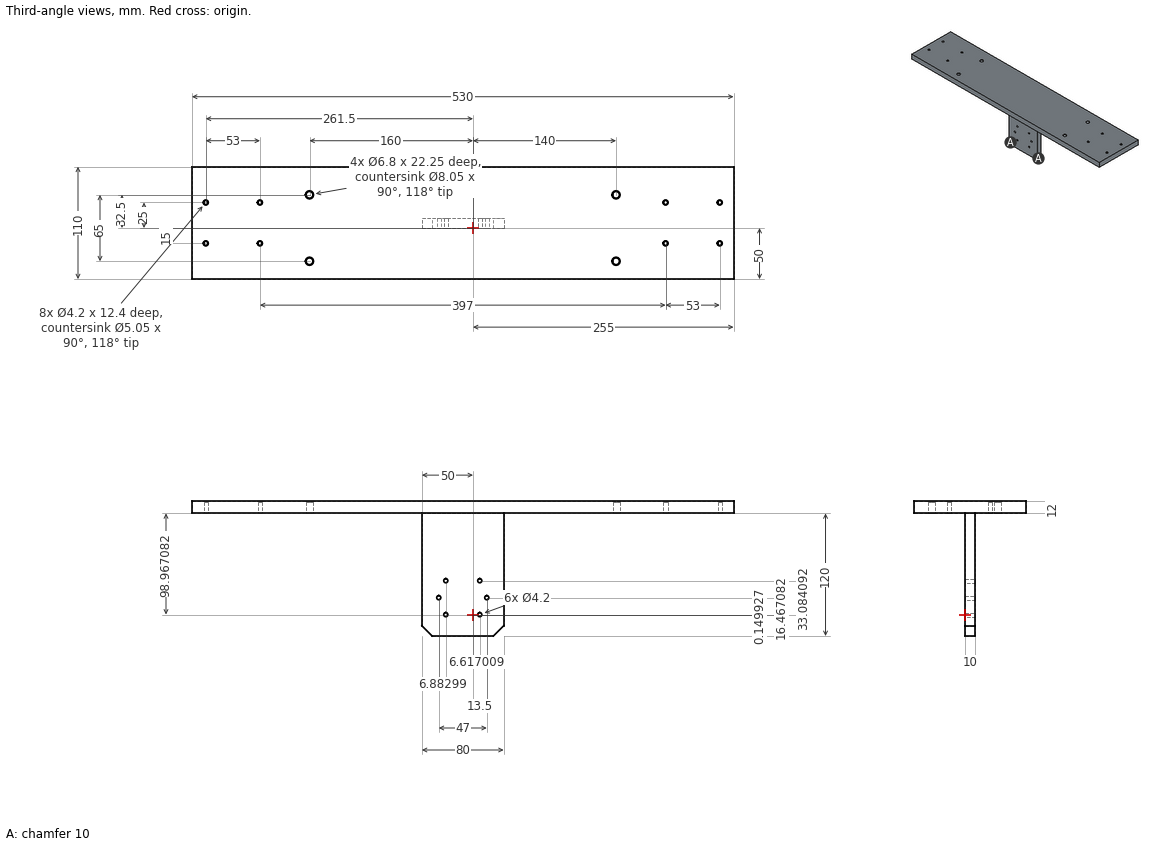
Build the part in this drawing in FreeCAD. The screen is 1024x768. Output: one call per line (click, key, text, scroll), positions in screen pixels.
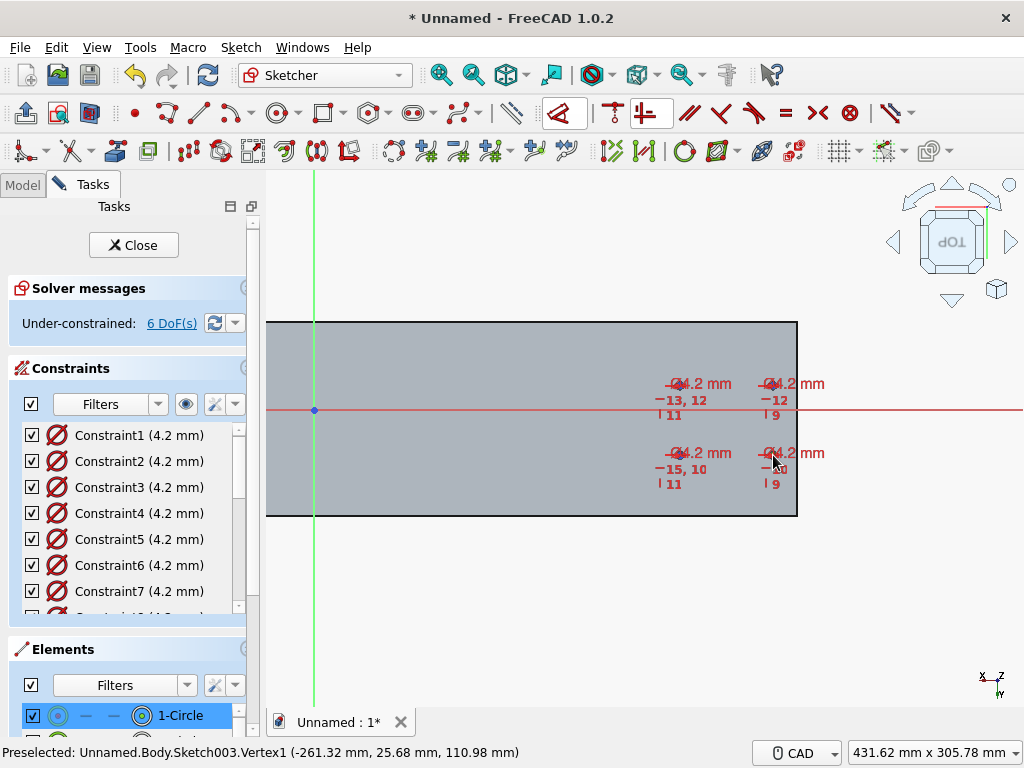
key(i)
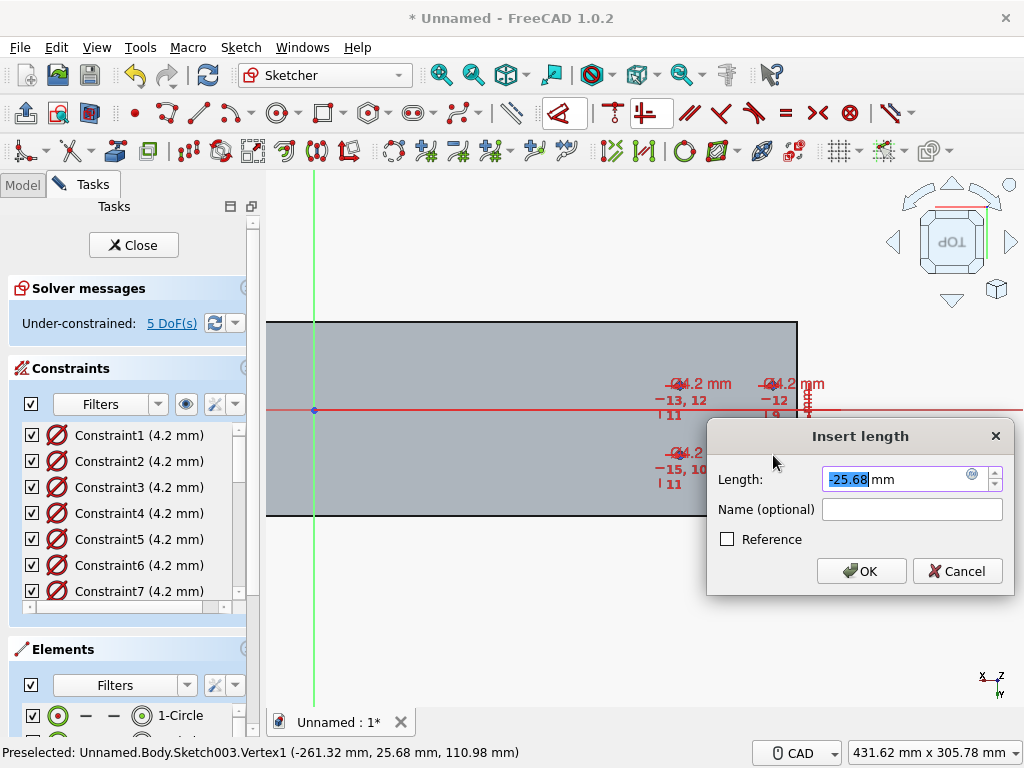
text(-25)
key(Return)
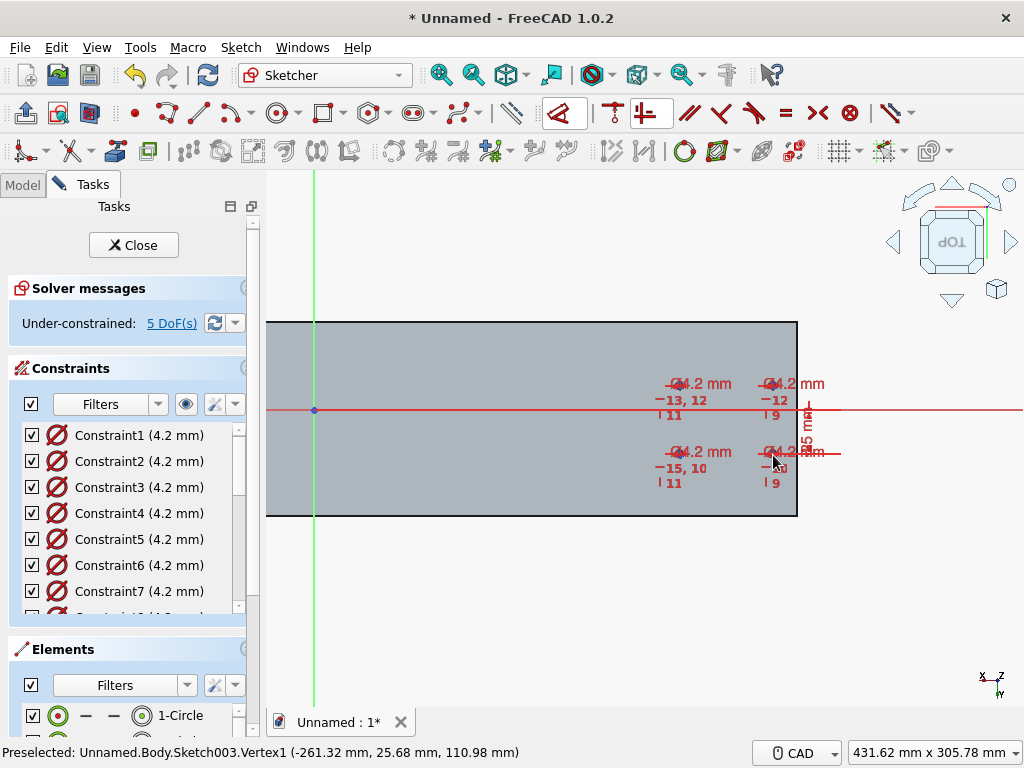
scroll(773, 386, up, 3)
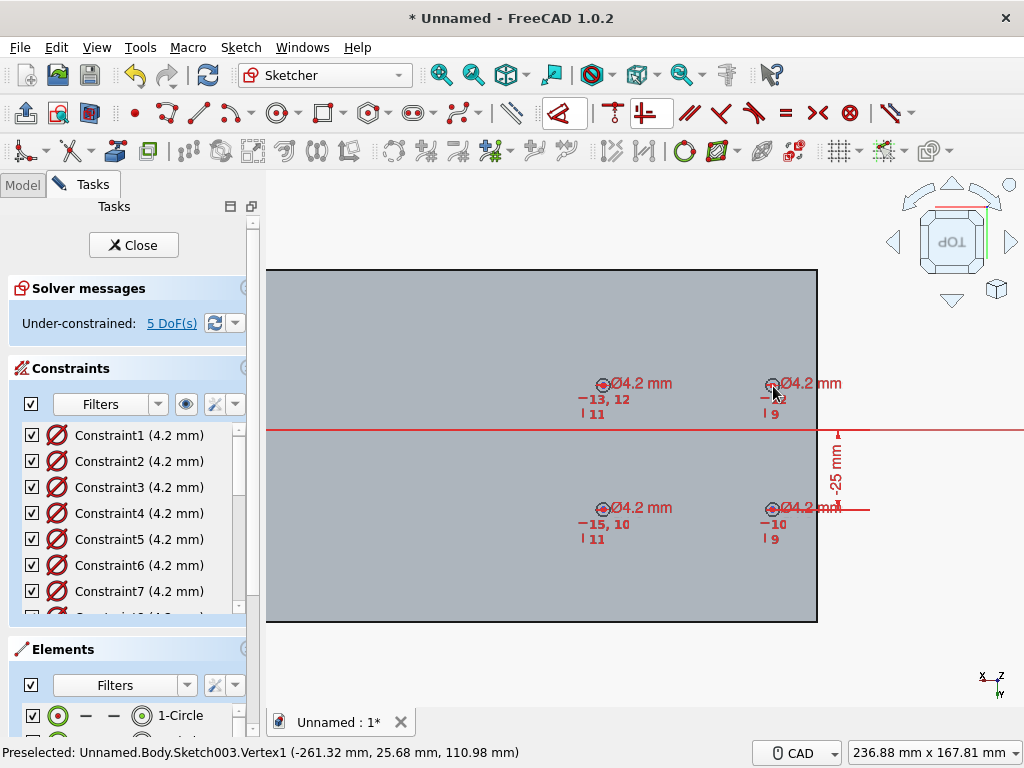
click(773, 385)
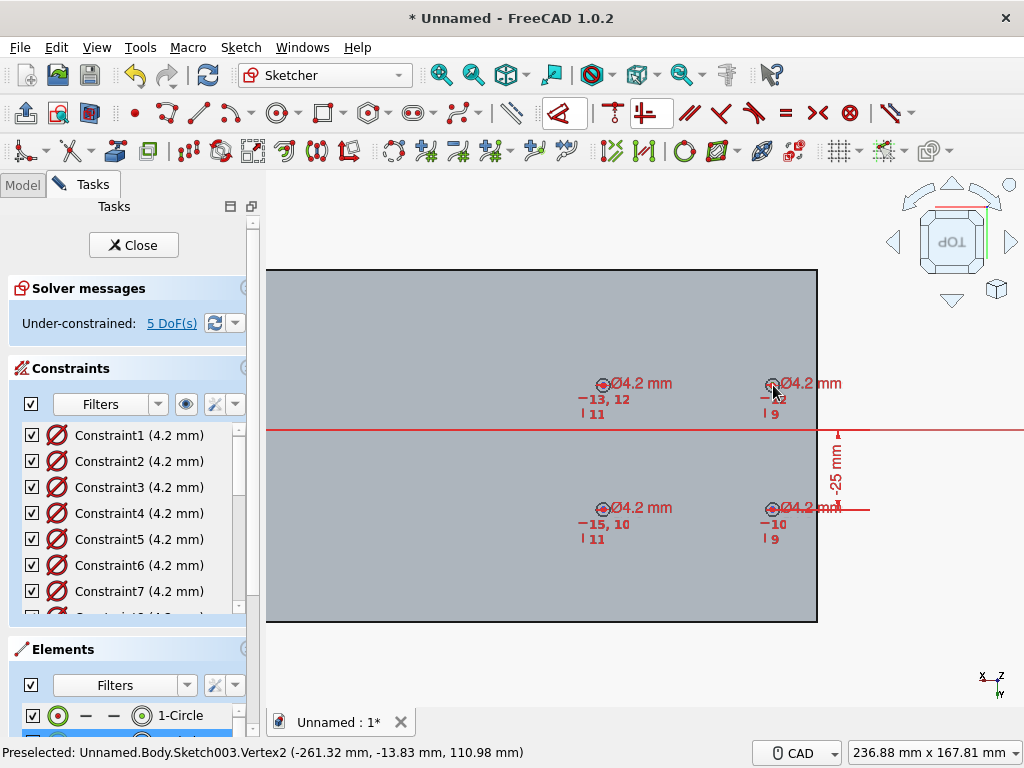
key(i)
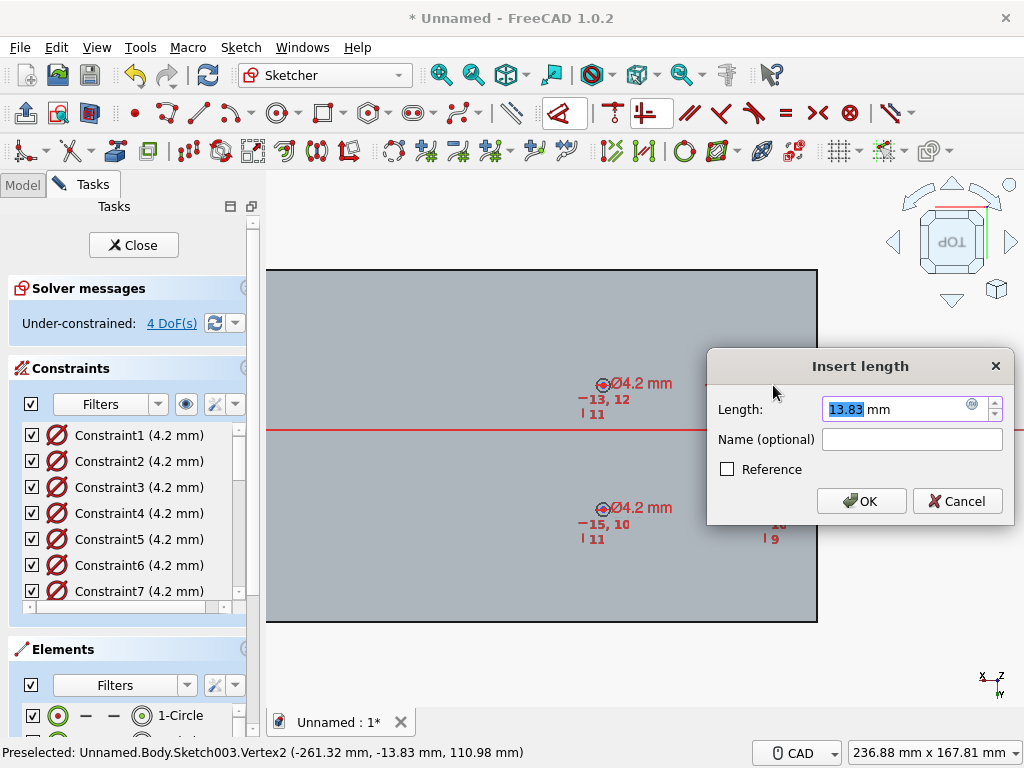
text(15)
key(Return)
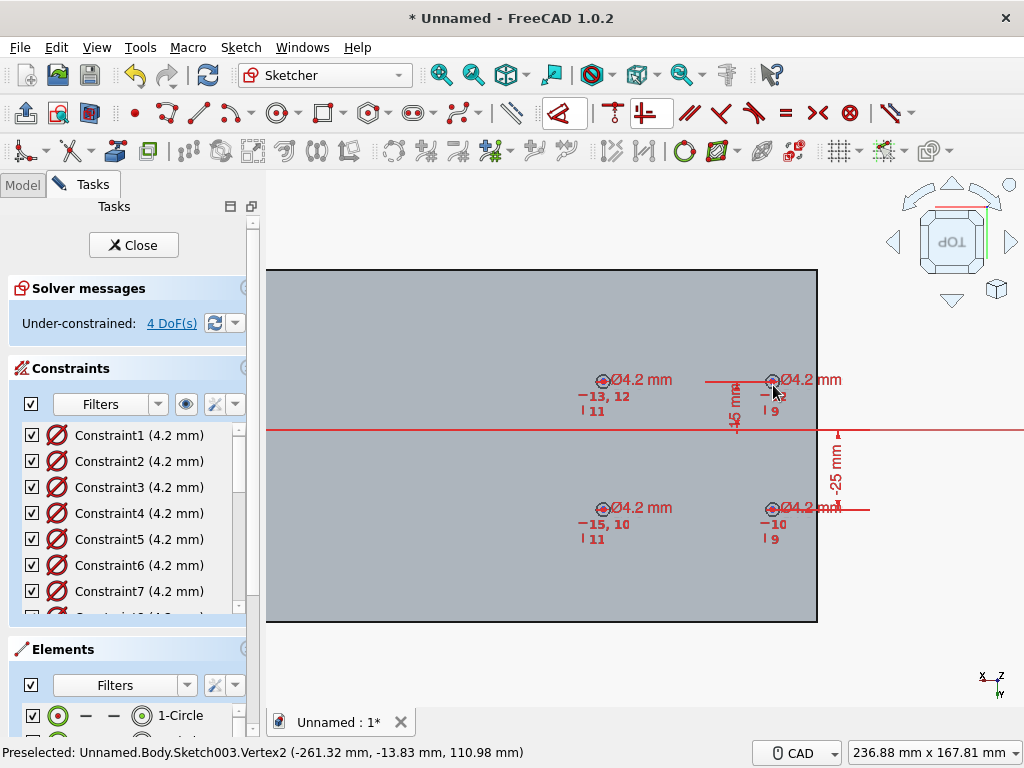
scroll(775, 436, down, 7)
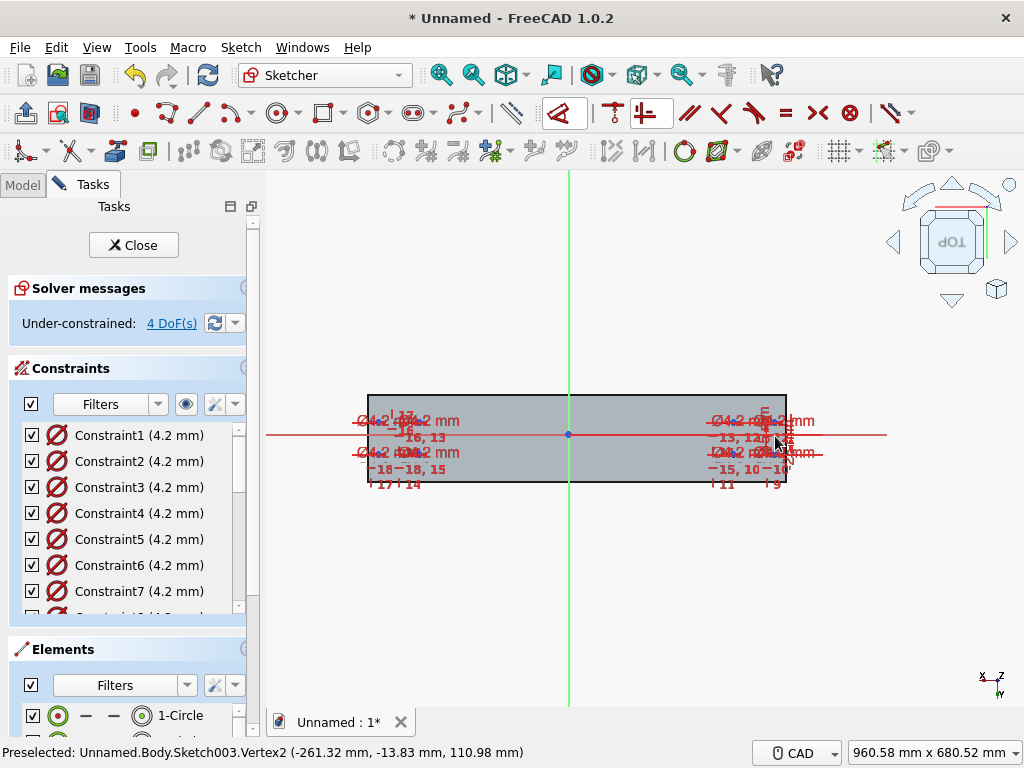
click(775, 455)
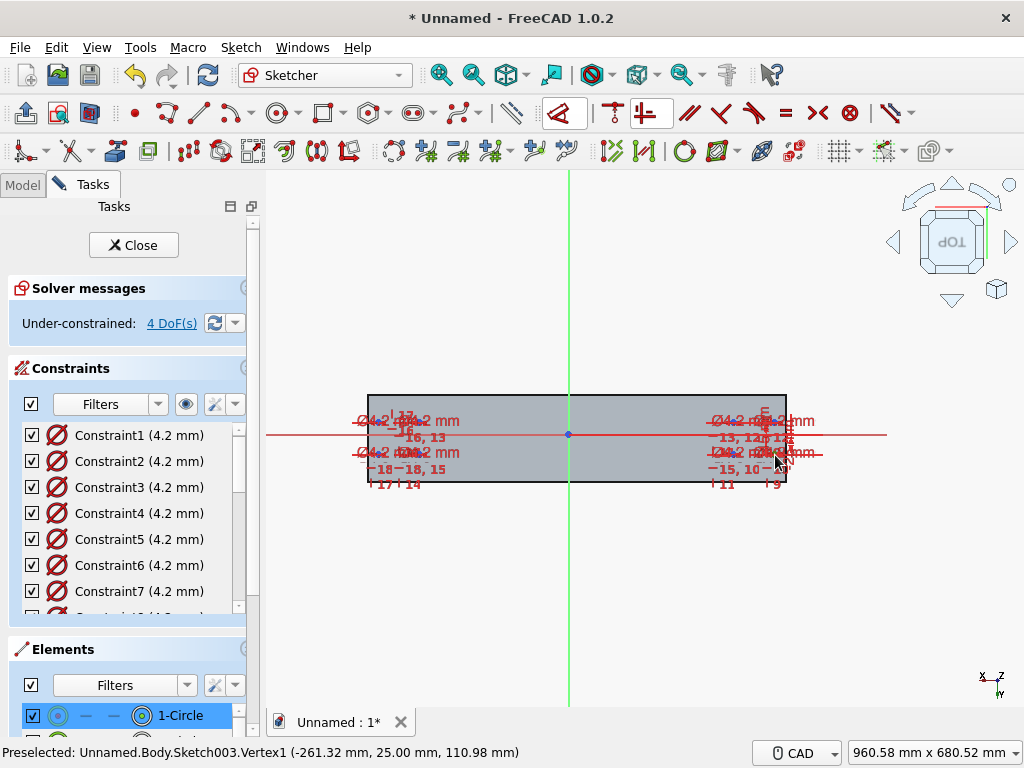
click(733, 455)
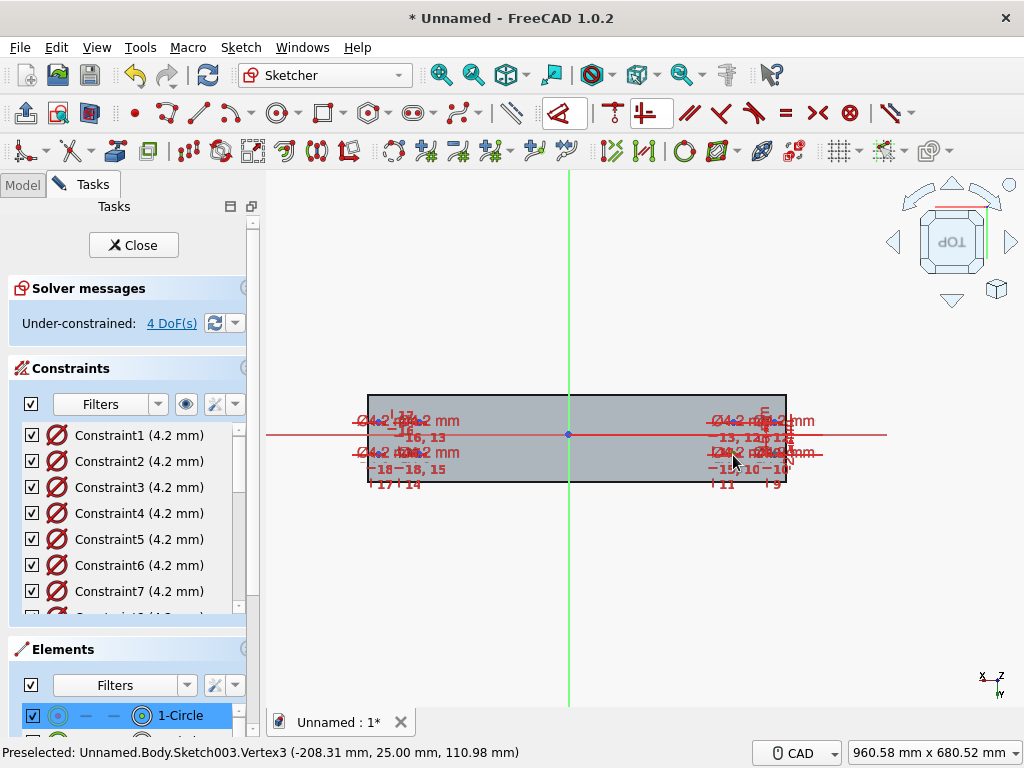
key(l)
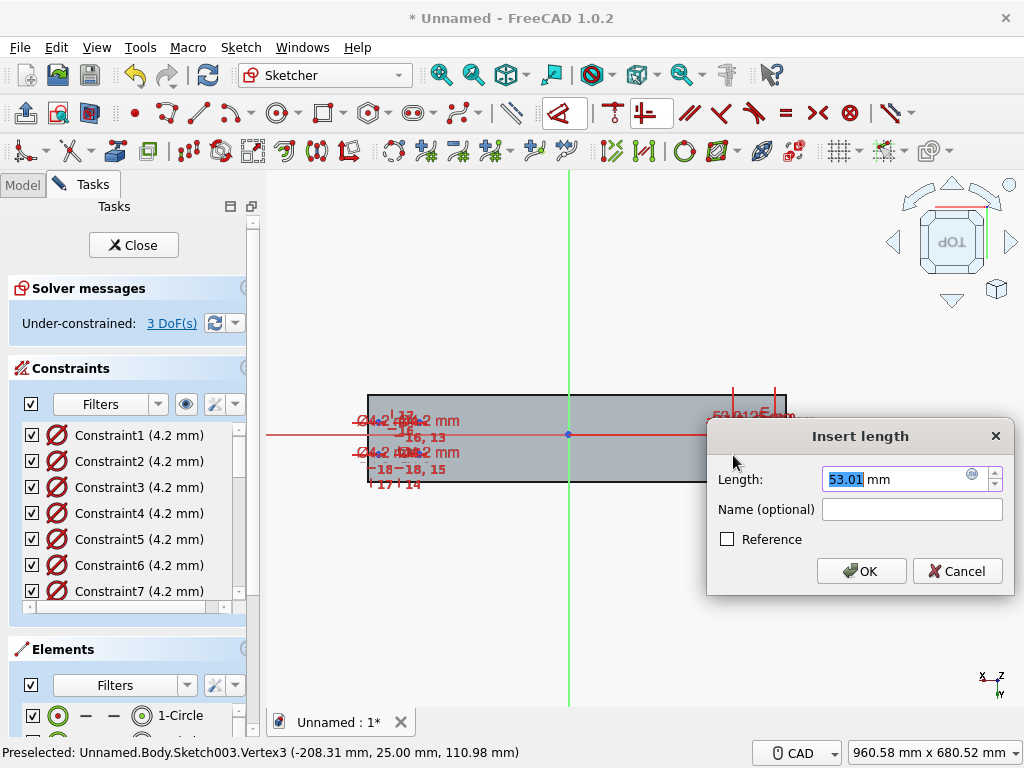
text(53)
key(Return)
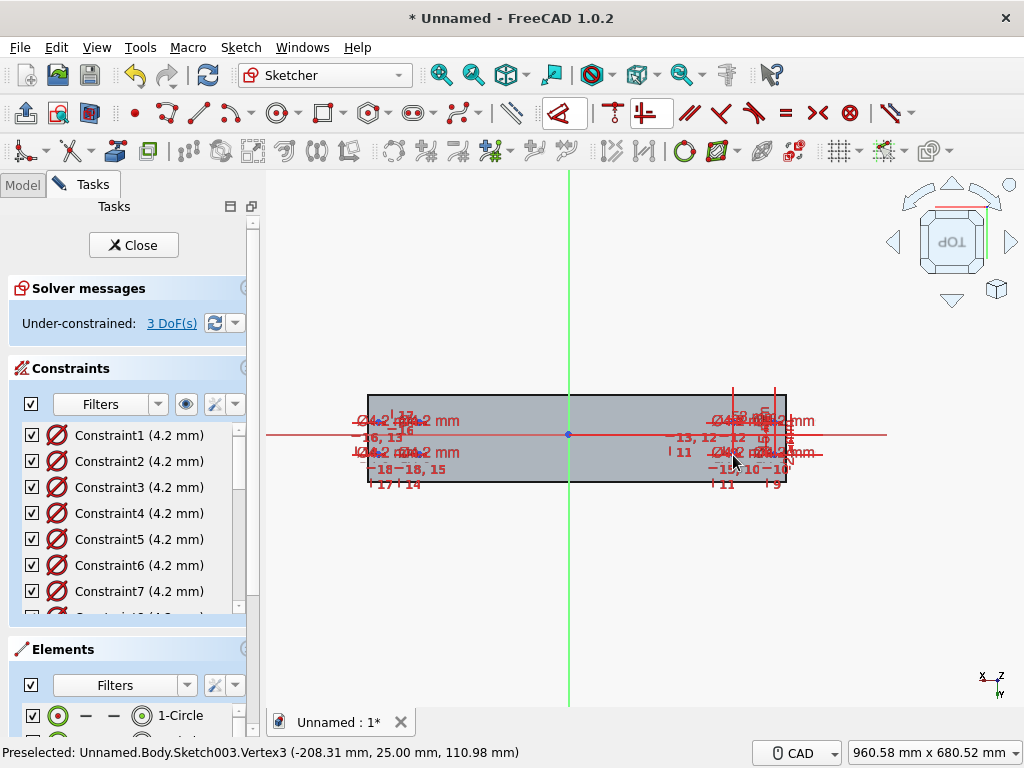
click(420, 423)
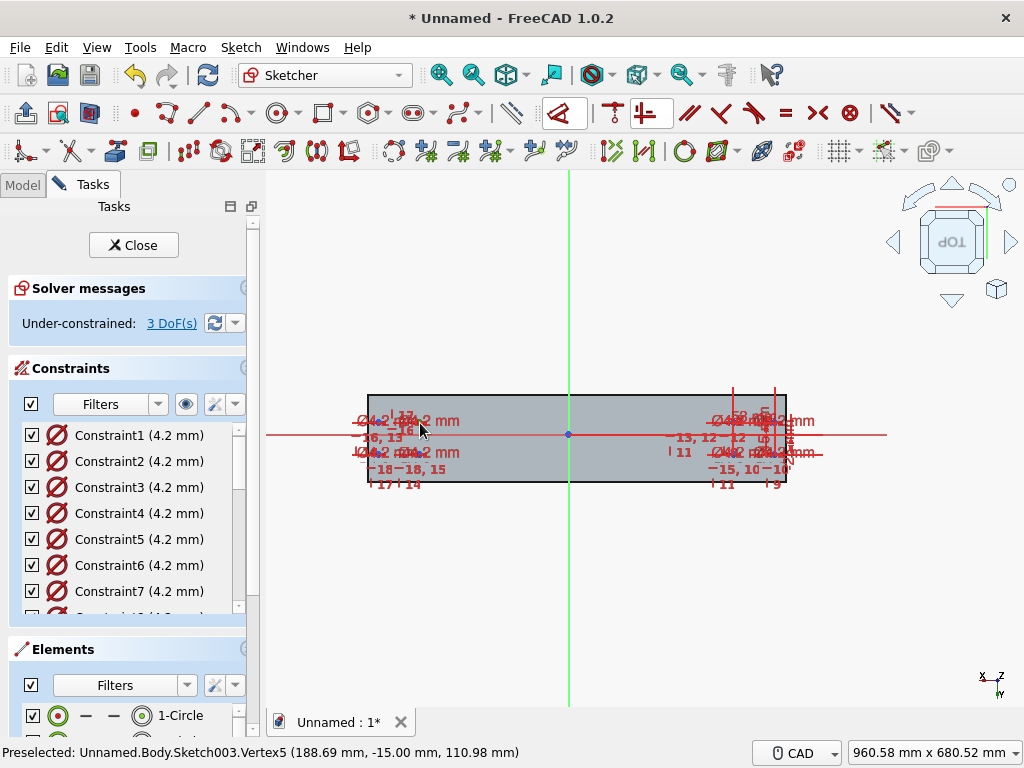
click(379, 423)